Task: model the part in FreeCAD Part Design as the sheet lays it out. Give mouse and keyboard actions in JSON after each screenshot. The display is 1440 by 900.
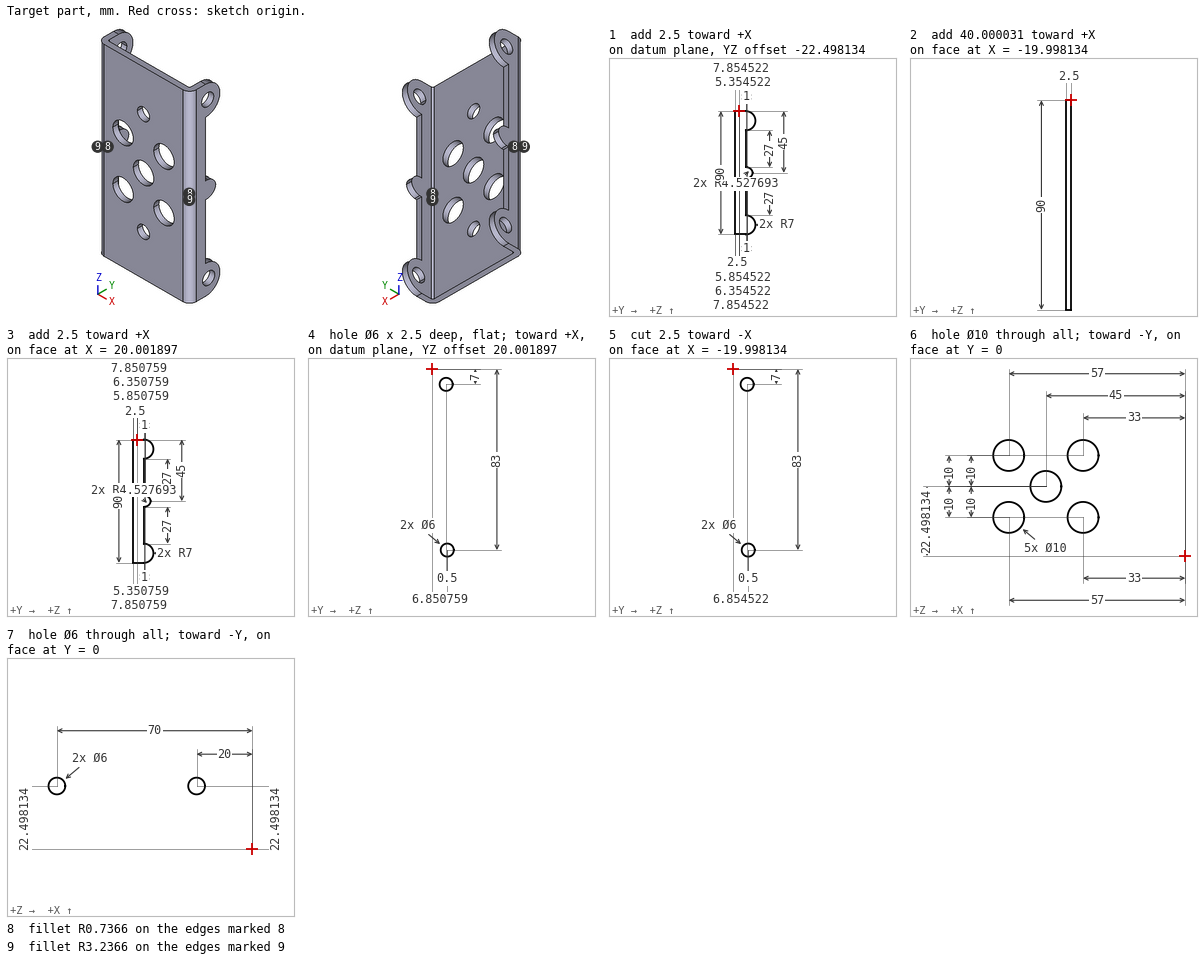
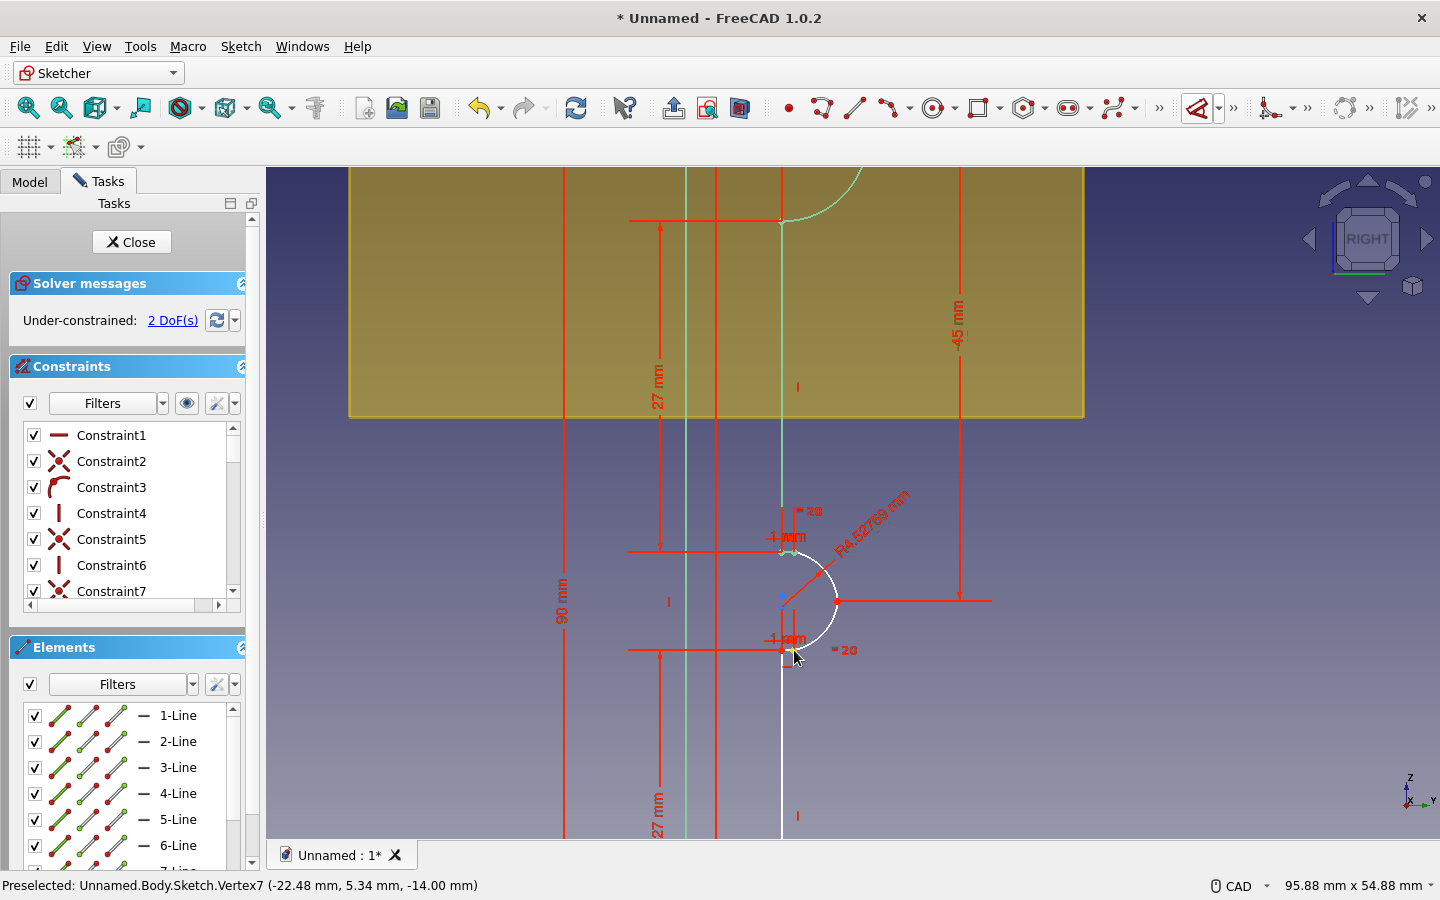
{"action": "left_click", "coordinate": [794, 650]}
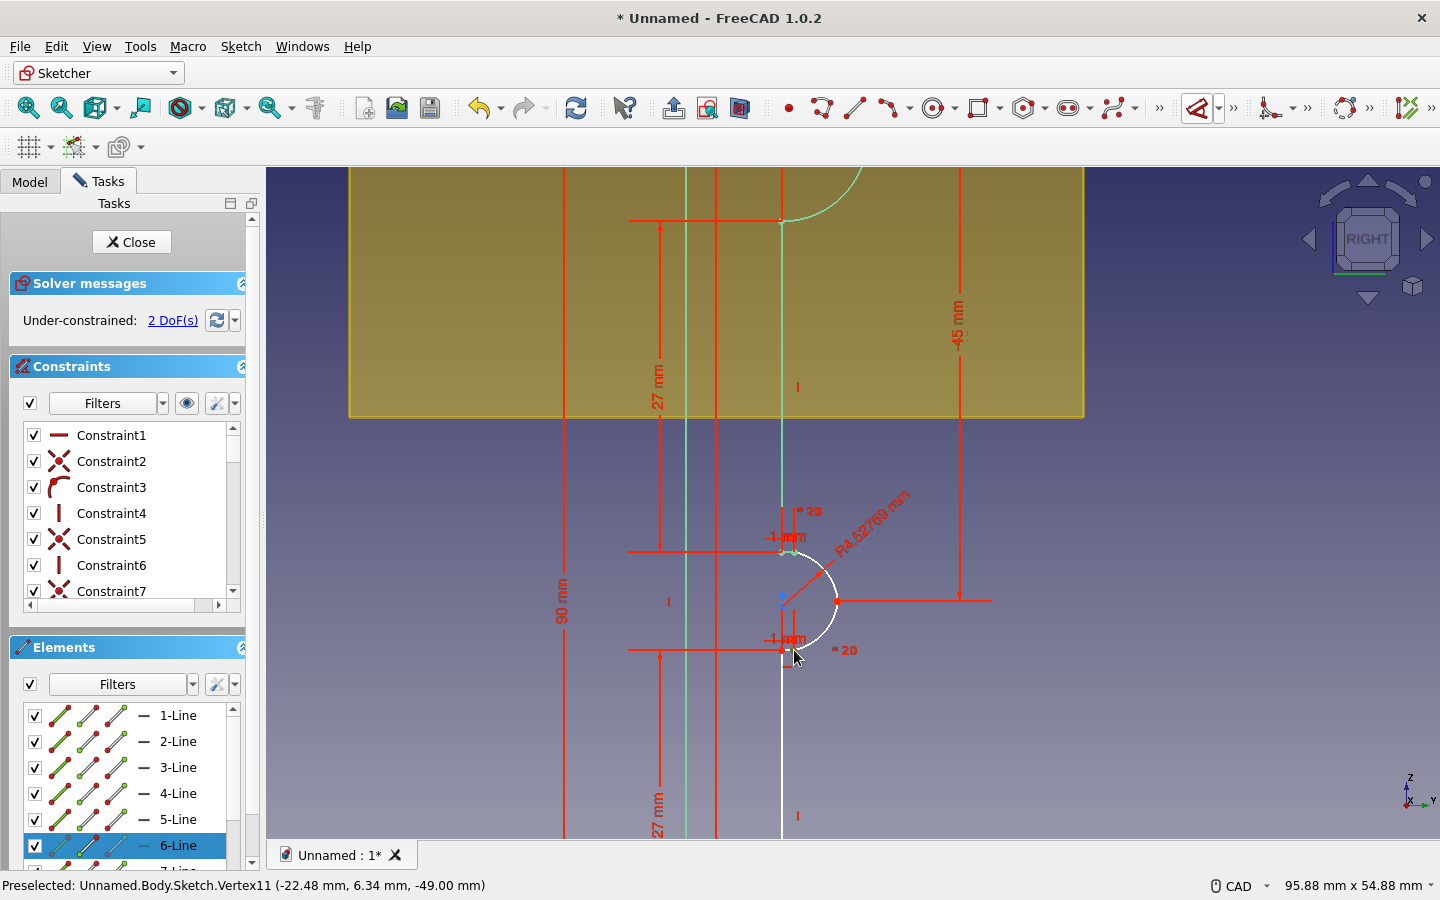
{"action": "key", "text": "l"}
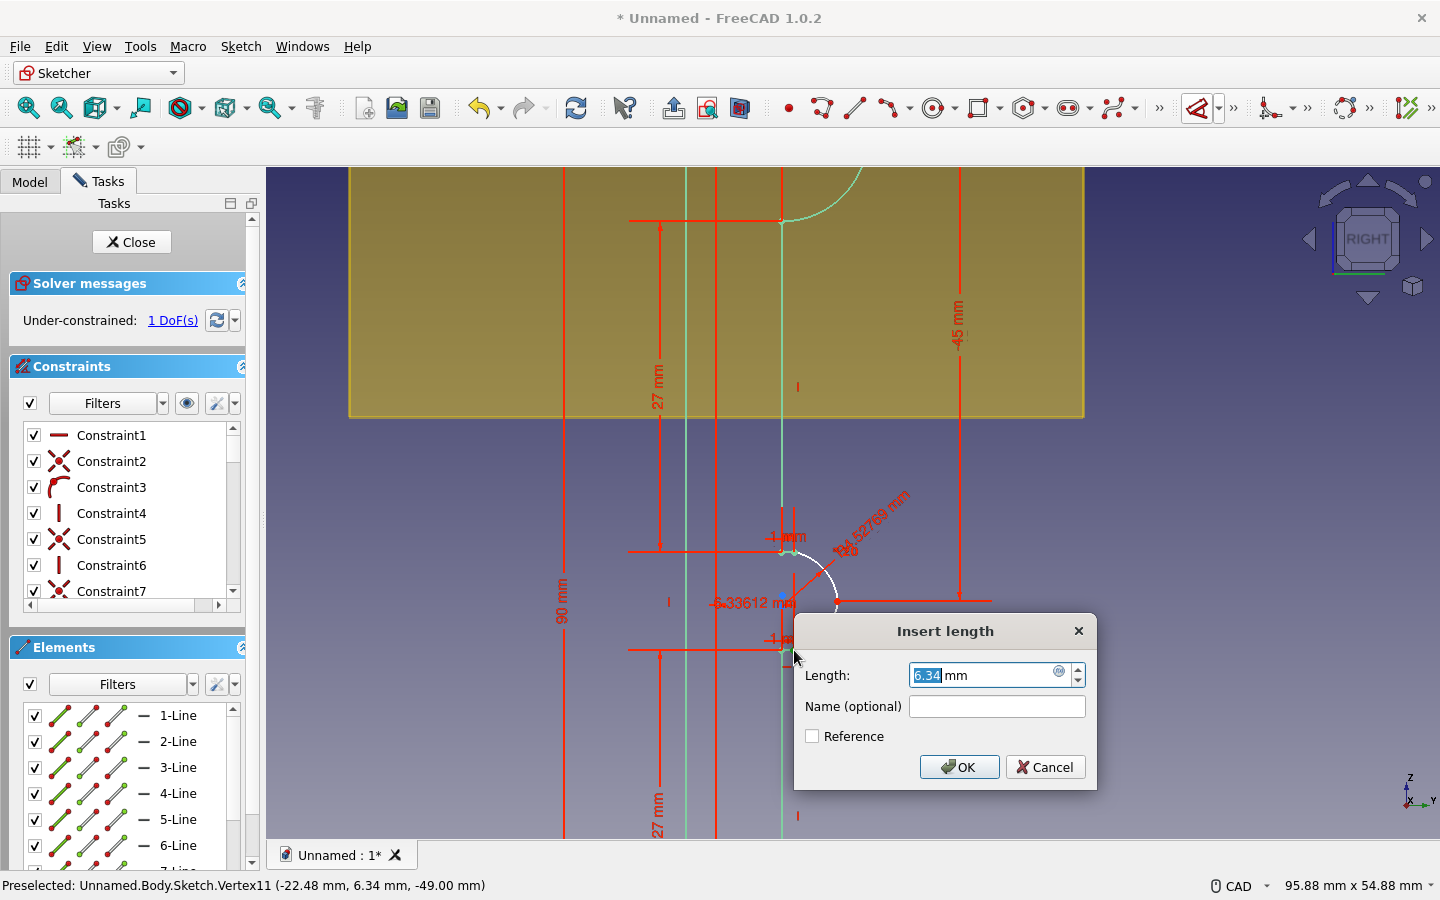
{"action": "type", "text": "6.354522"}
{"action": "key", "text": "Return"}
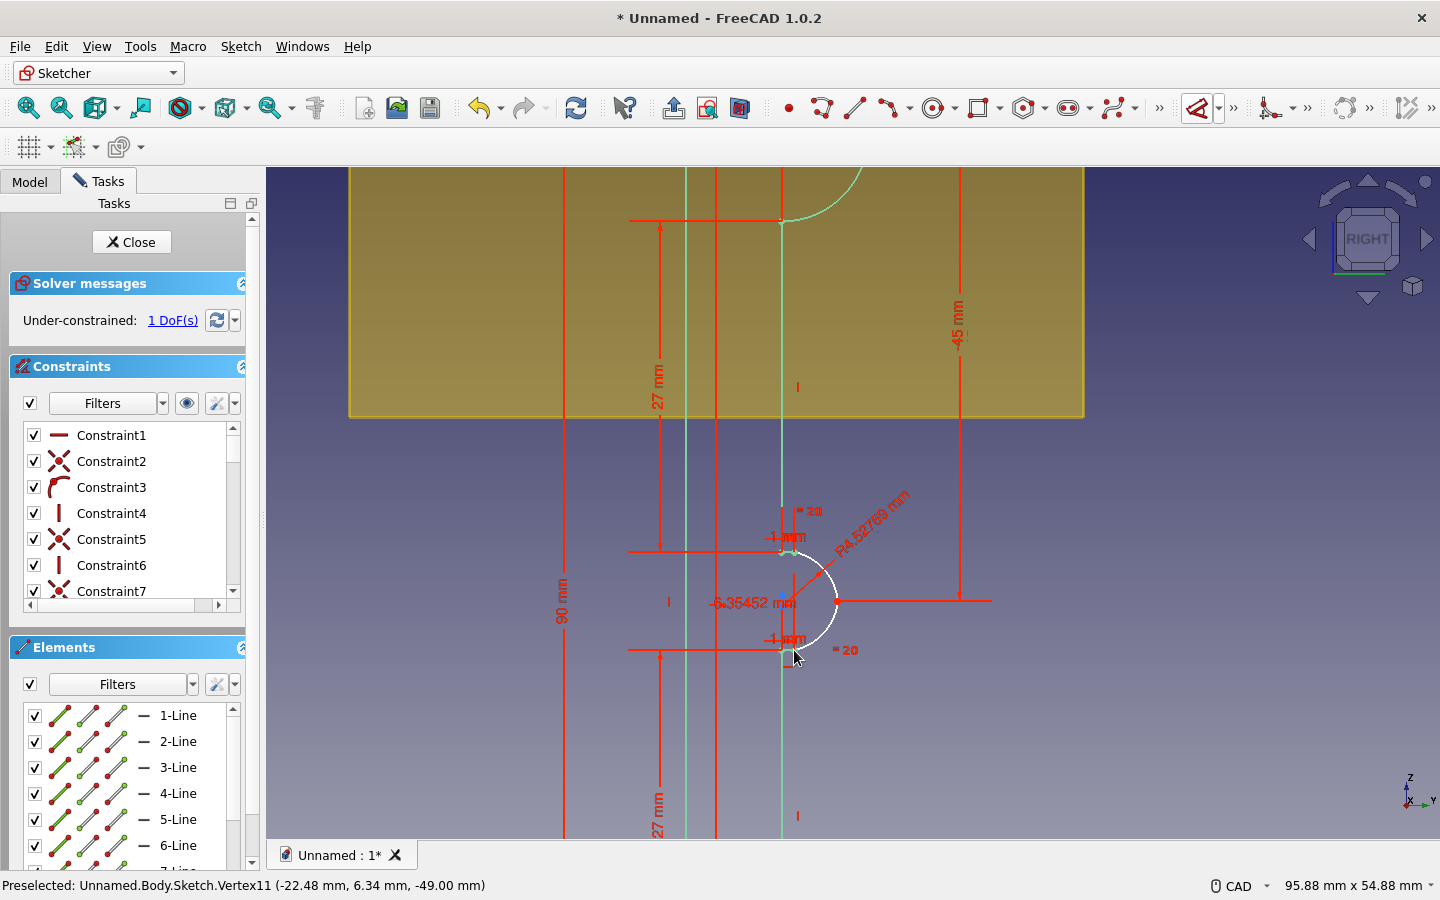
{"action": "left_click", "coordinate": [783, 606]}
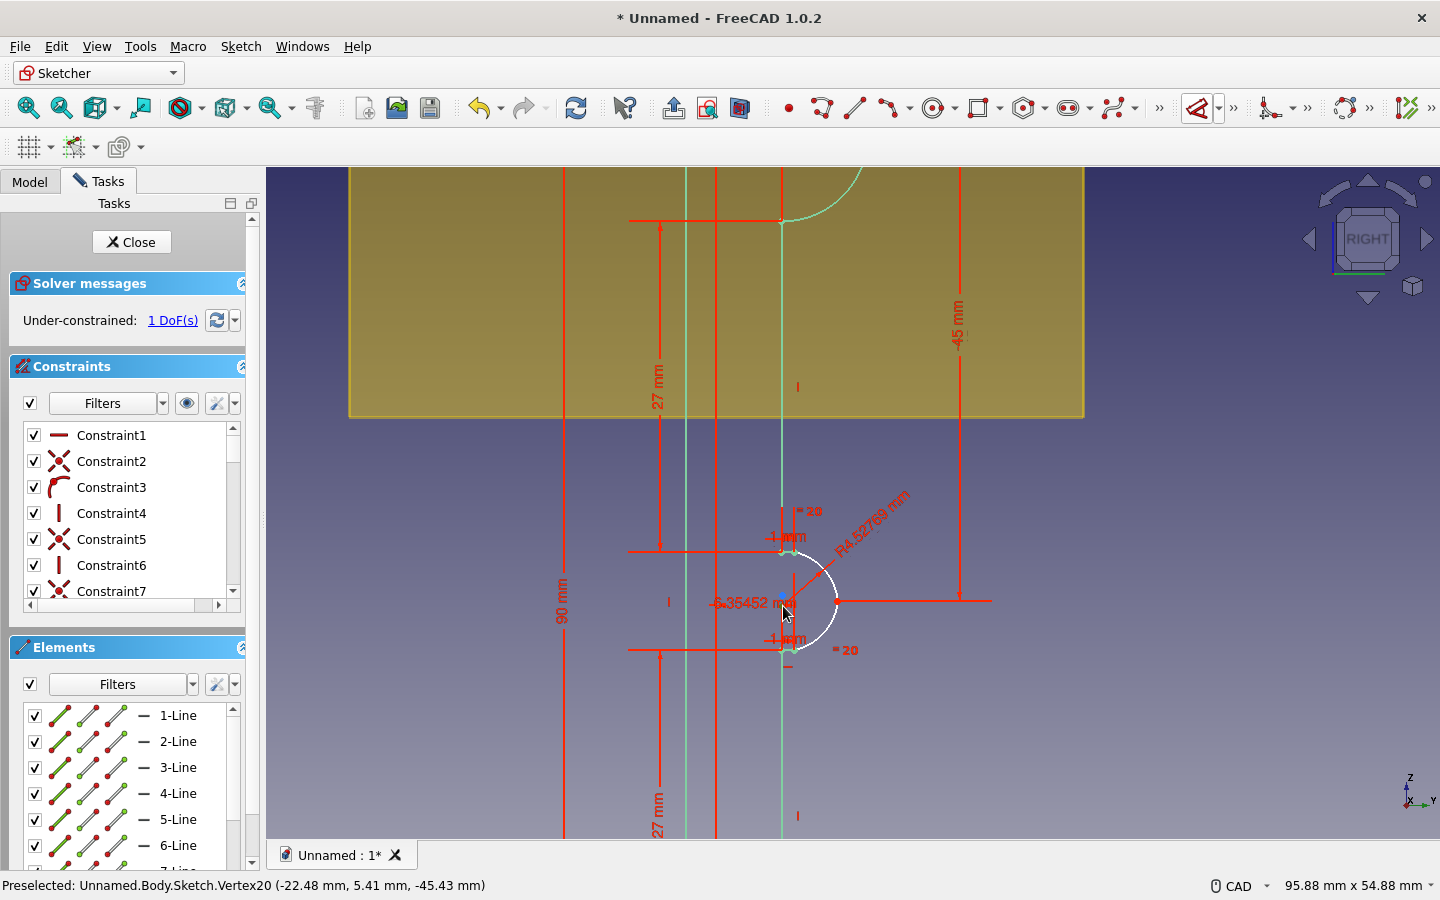
{"action": "key", "text": "l"}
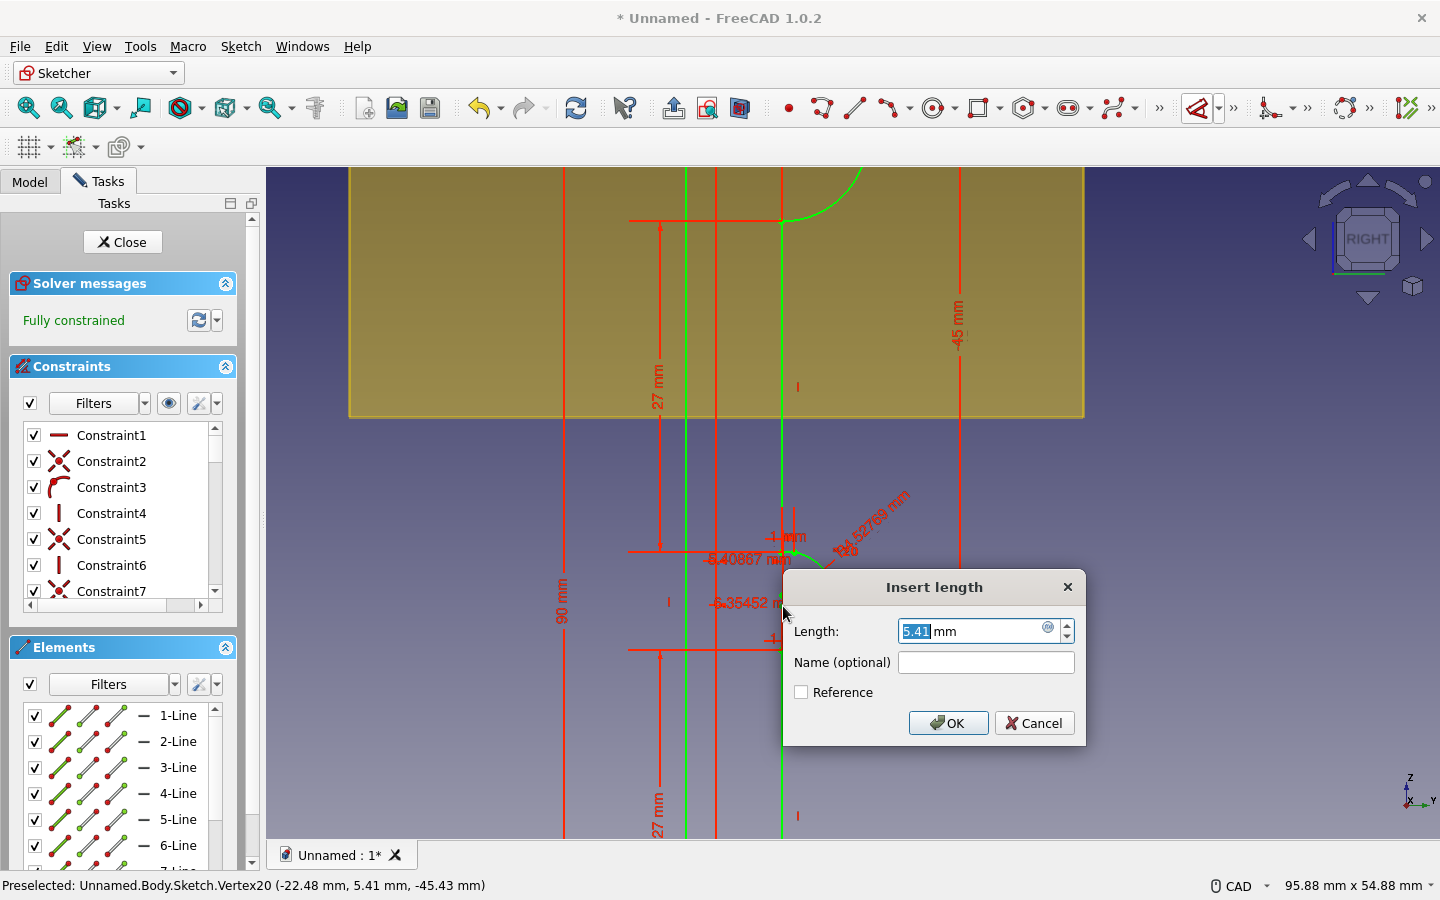
{"action": "type", "text": "5.854522"}
{"action": "key", "text": "Return"}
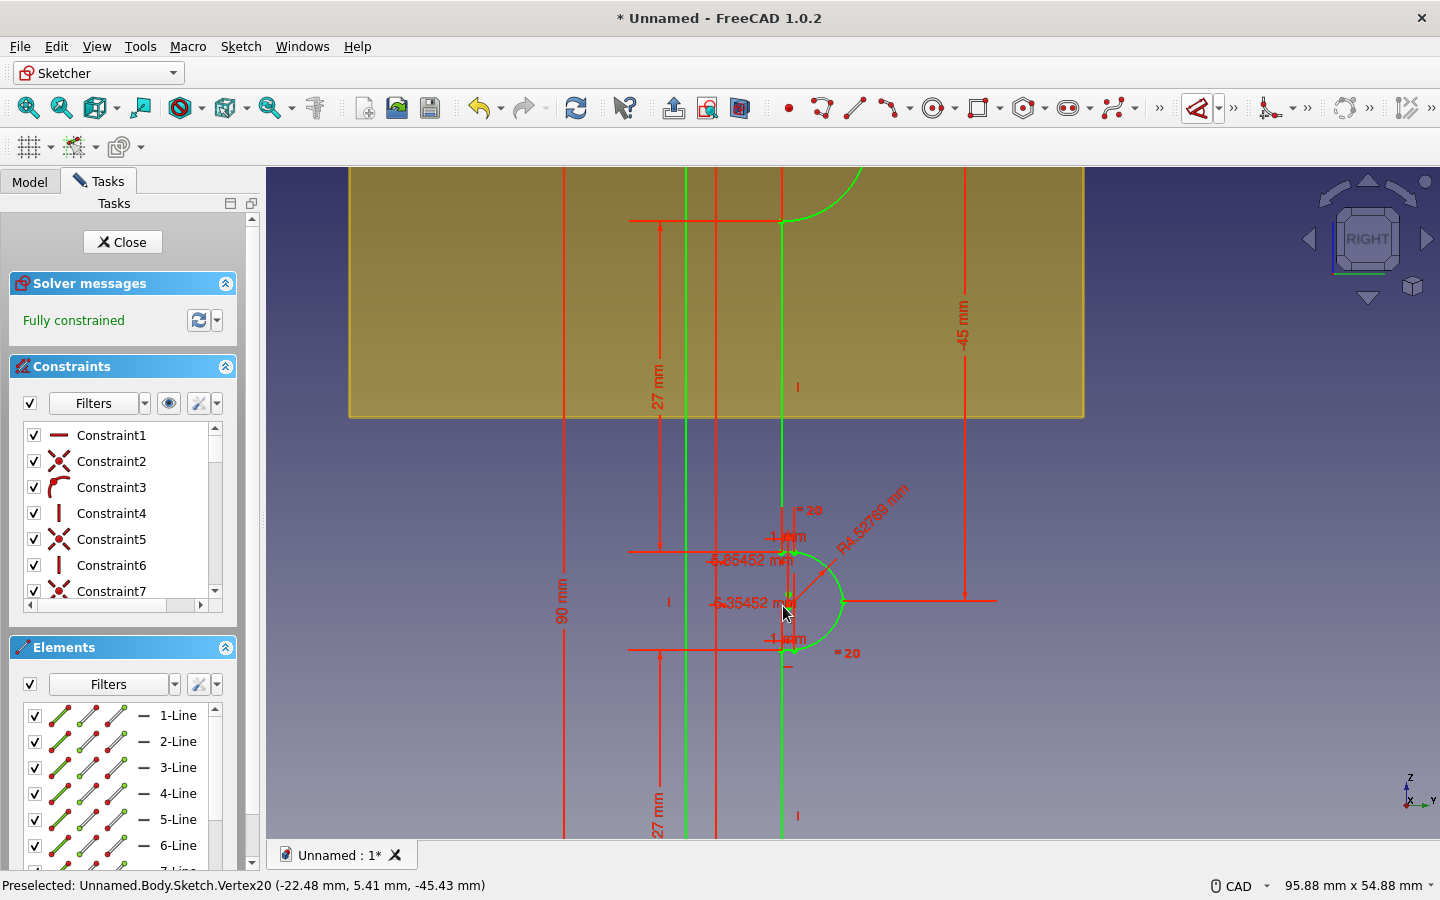
{"action": "left_click", "coordinate": [123, 242]}